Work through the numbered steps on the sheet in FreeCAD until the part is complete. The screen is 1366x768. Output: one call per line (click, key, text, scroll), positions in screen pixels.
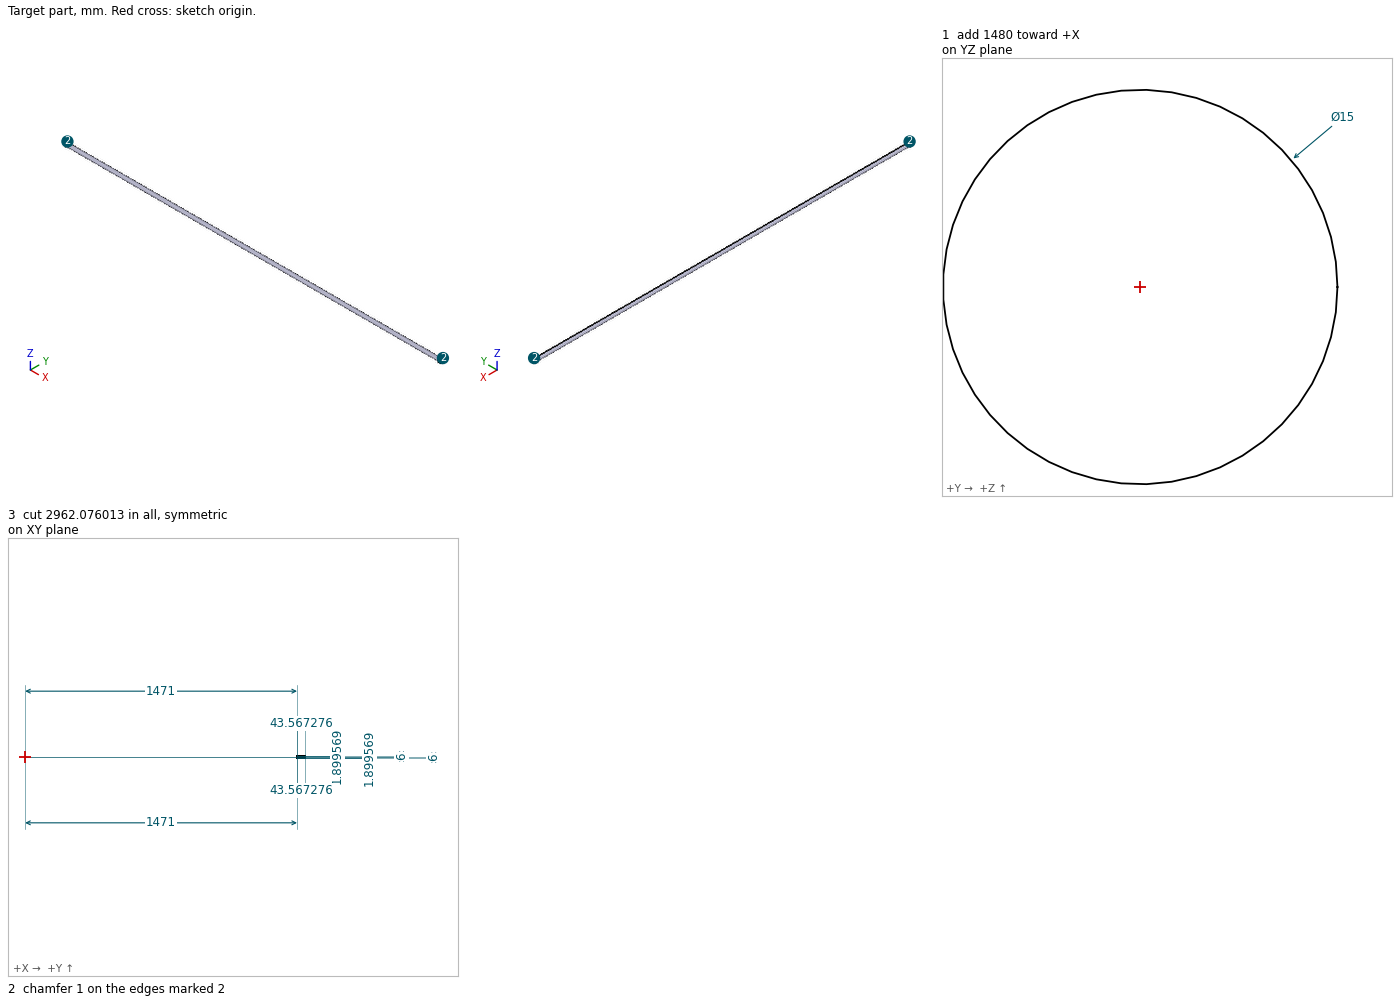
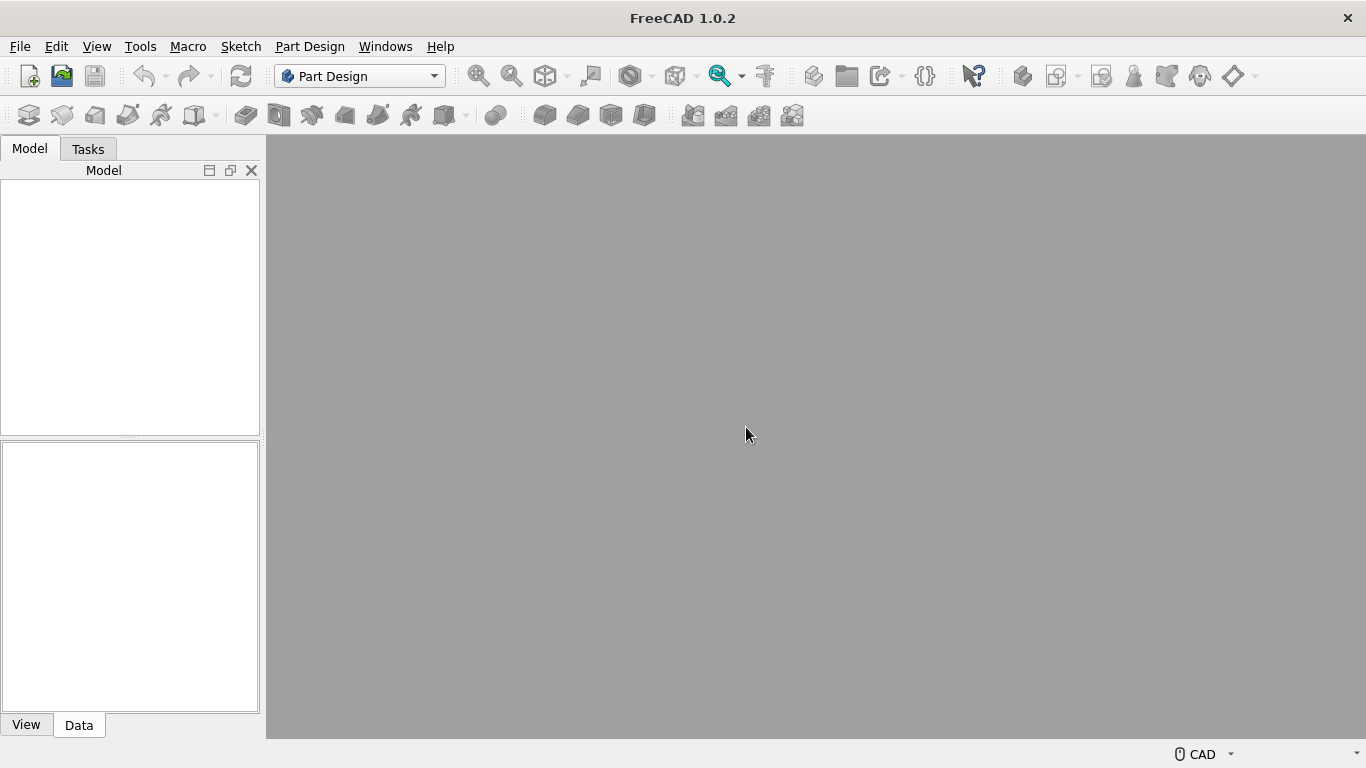
key(ctrl+n)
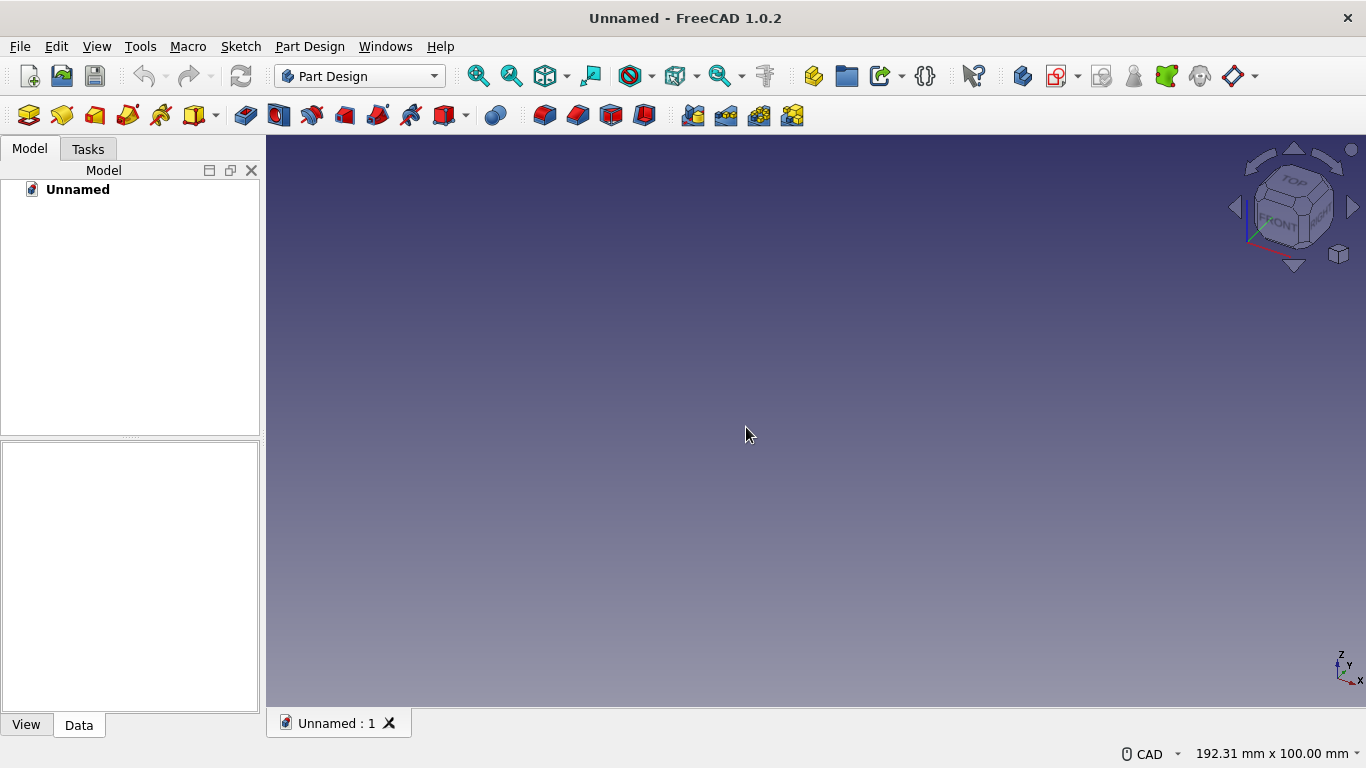
click(1056, 76)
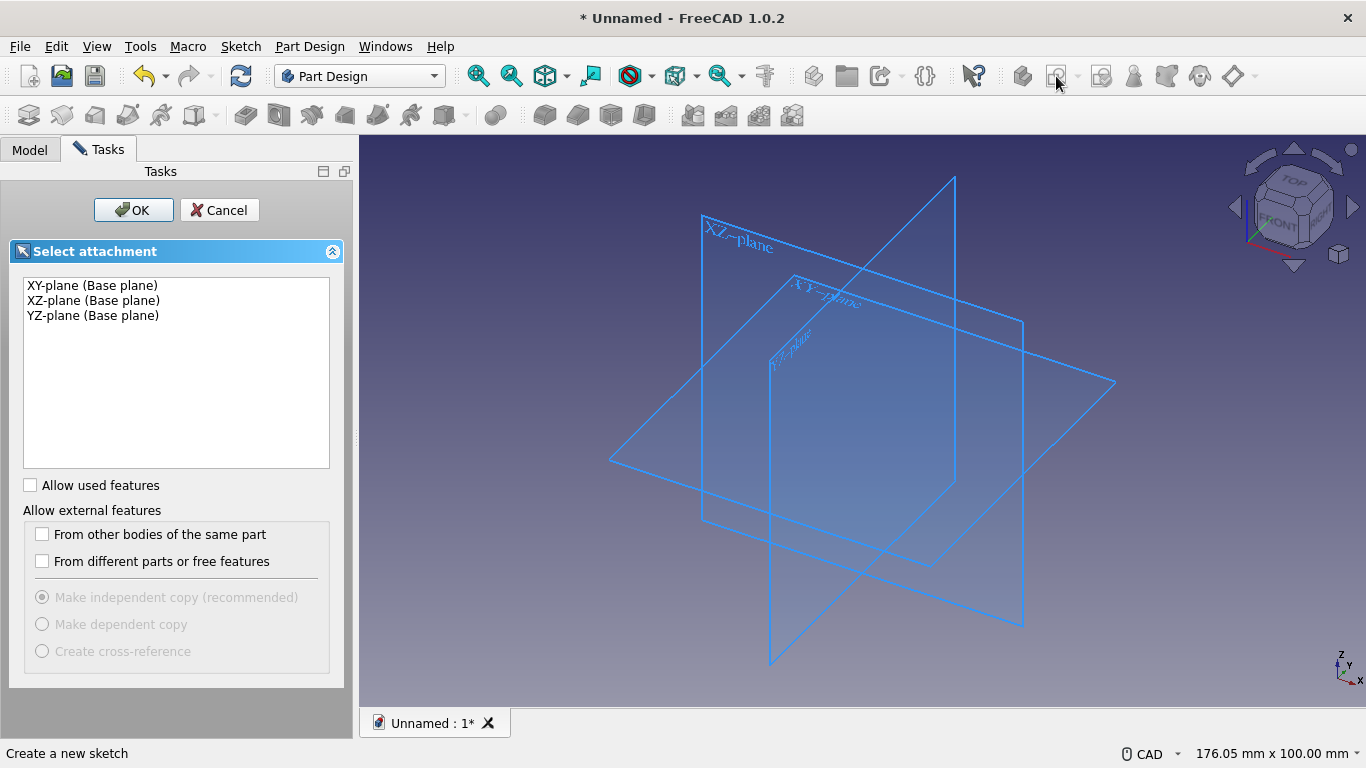
click(84, 316)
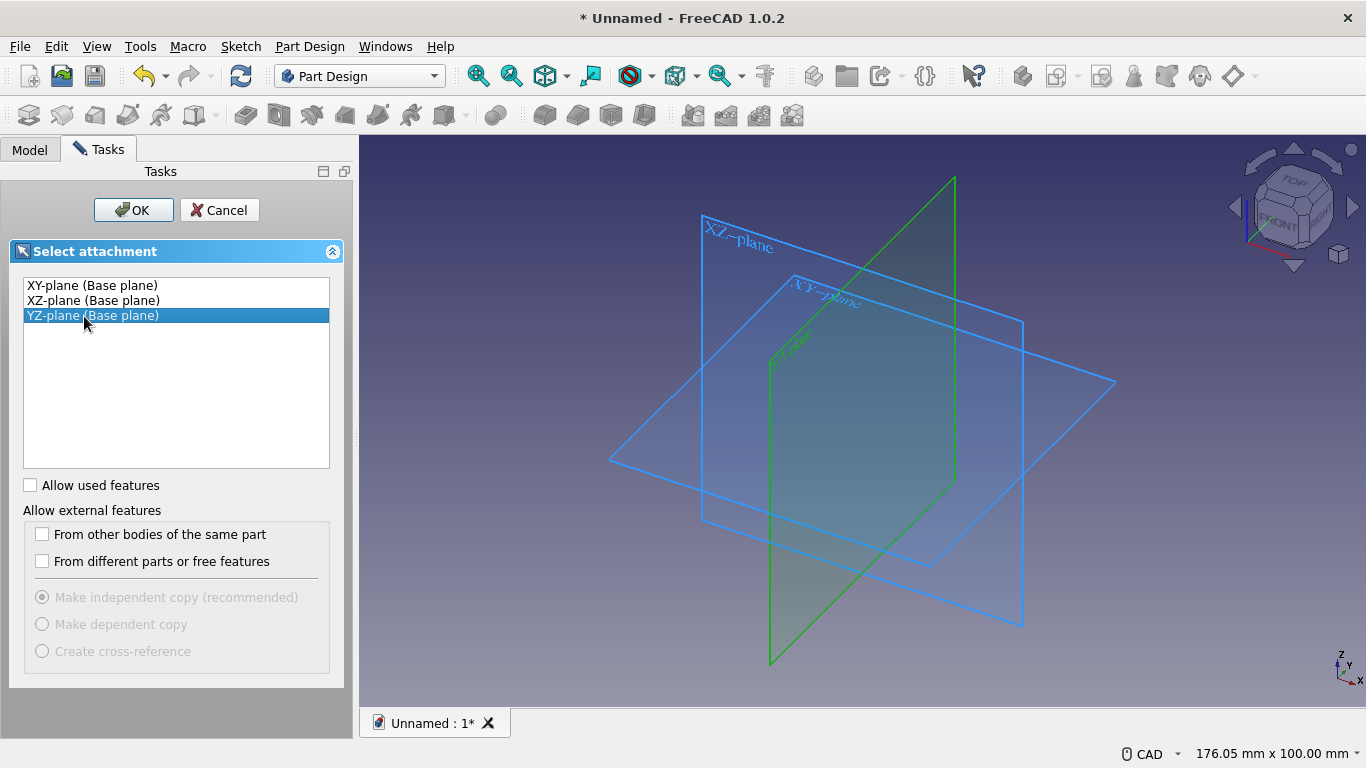
click(134, 210)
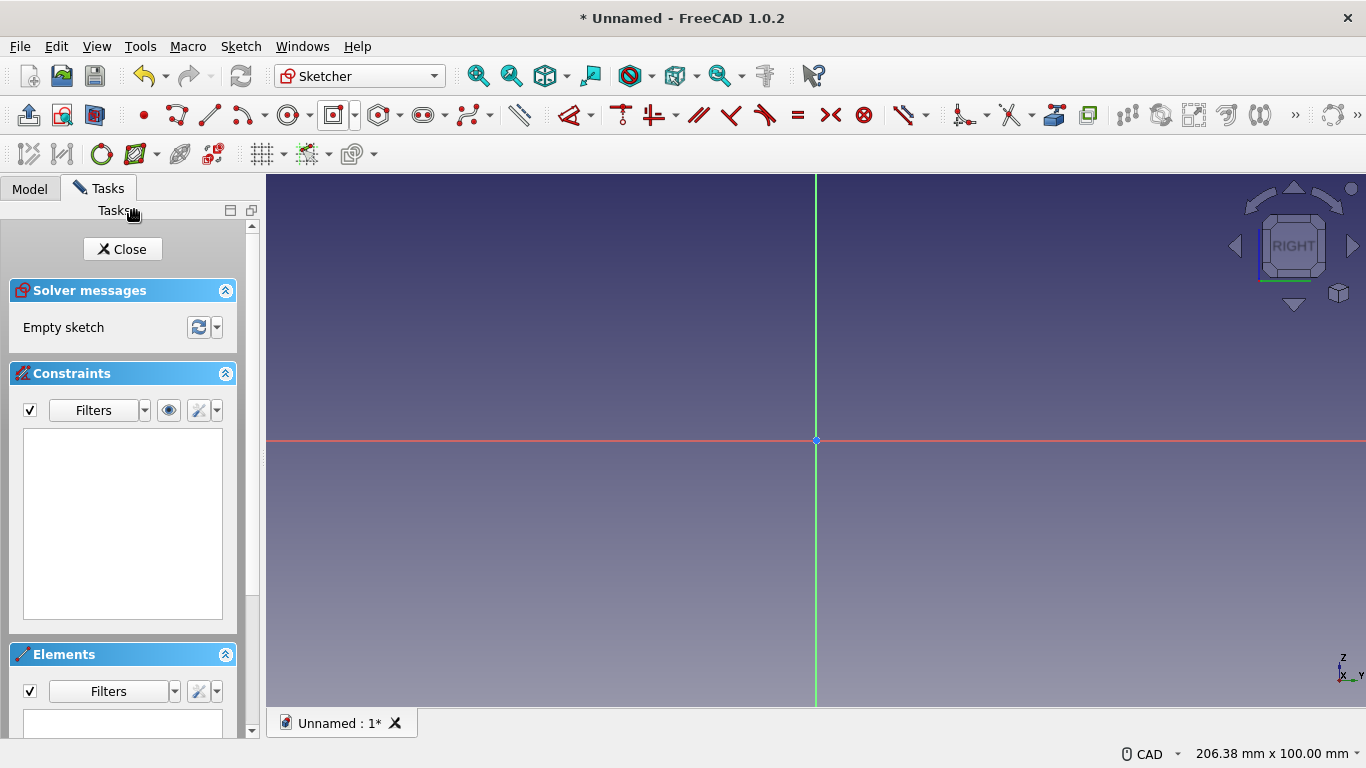
scroll(838, 440, up, 7)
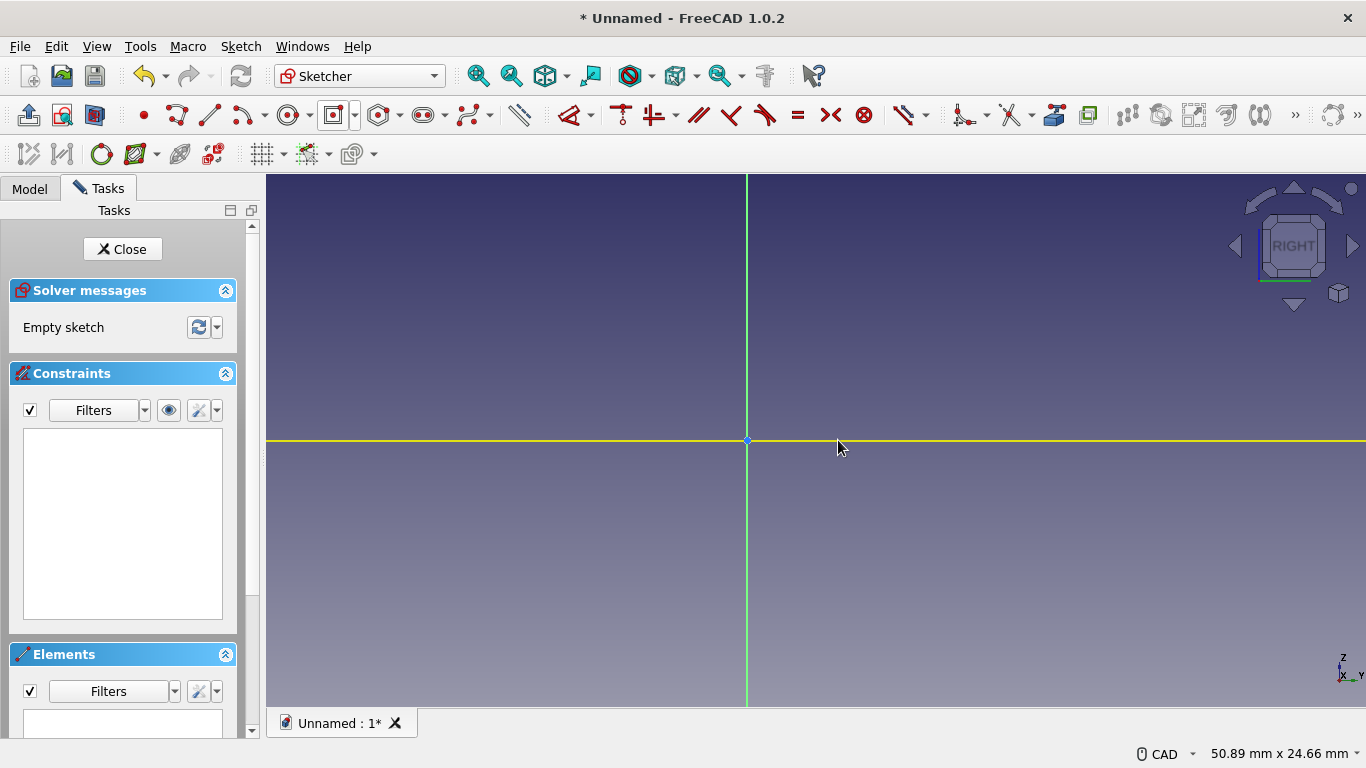
key(g)
key(c)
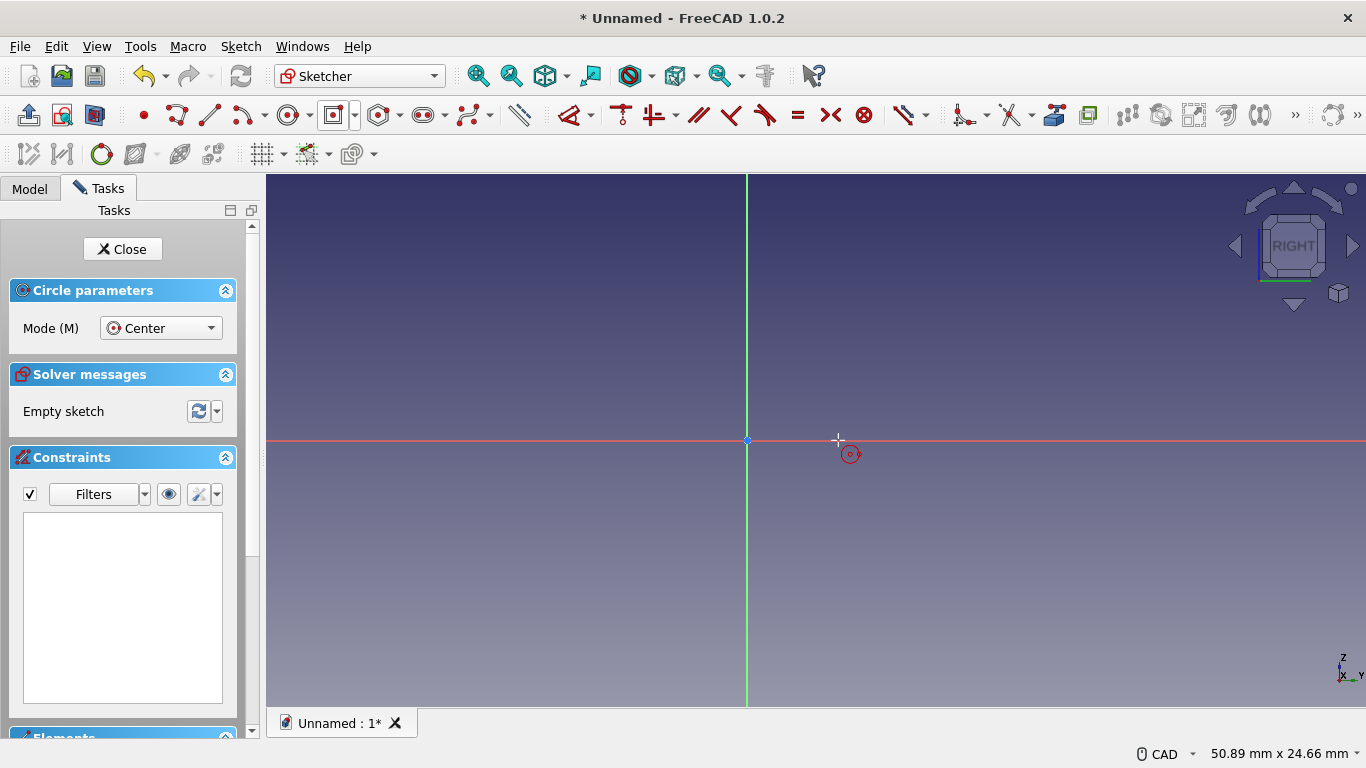
click(747, 440)
click(862, 326)
key(Escape)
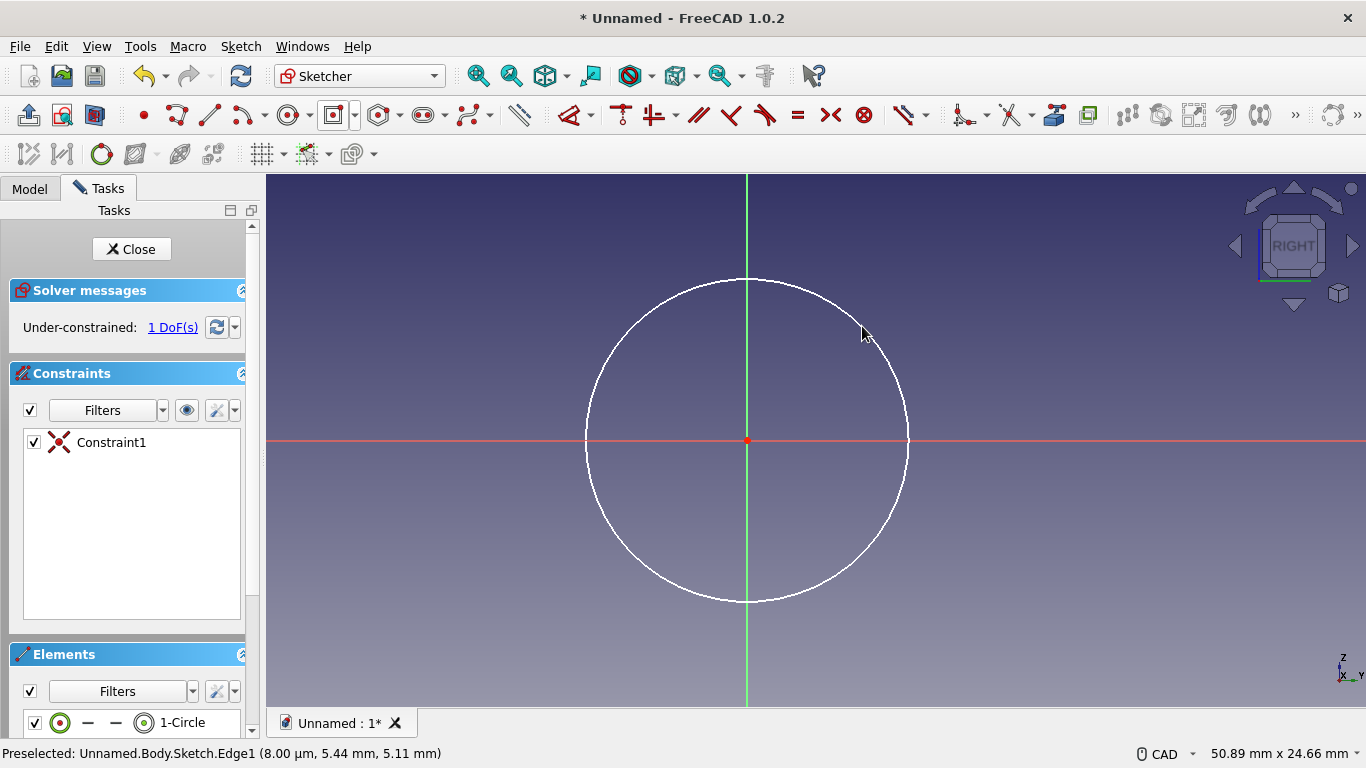
click(568, 116)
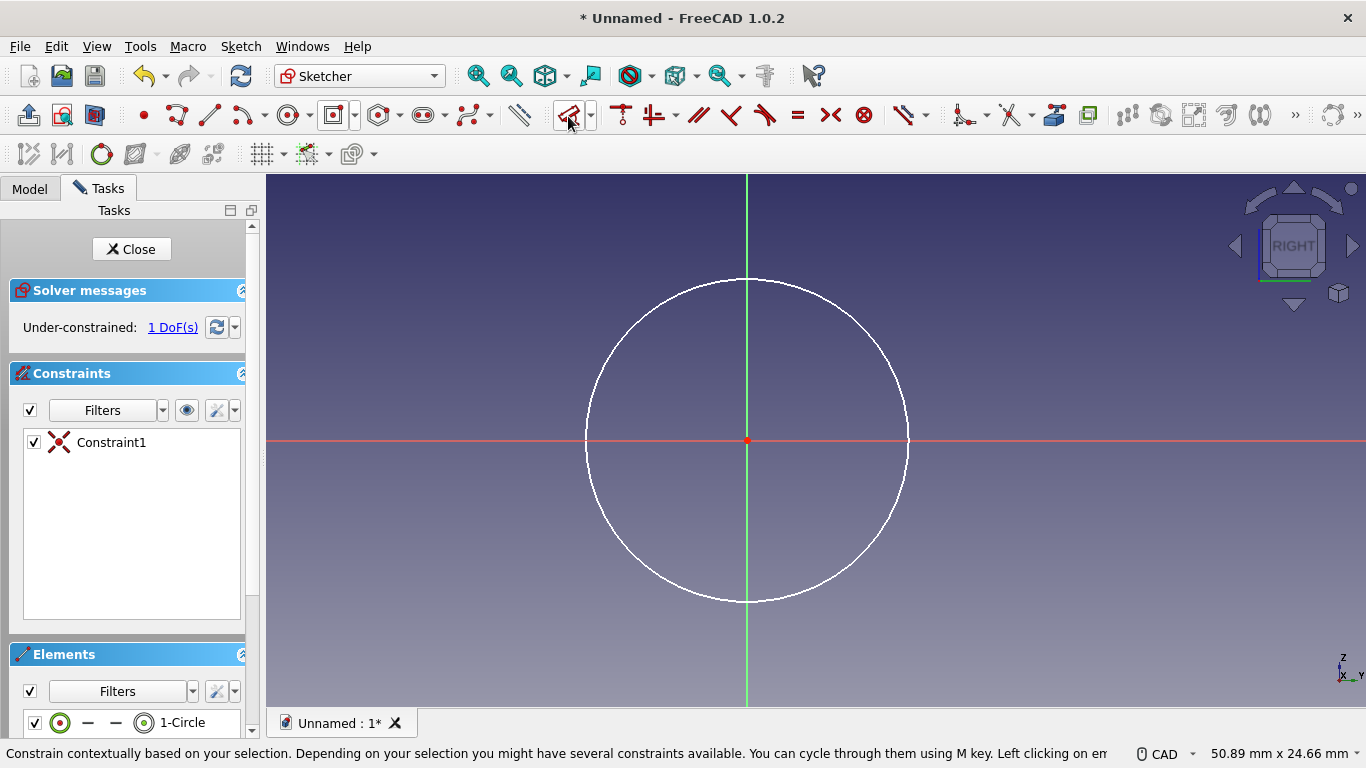
click(861, 326)
click(884, 303)